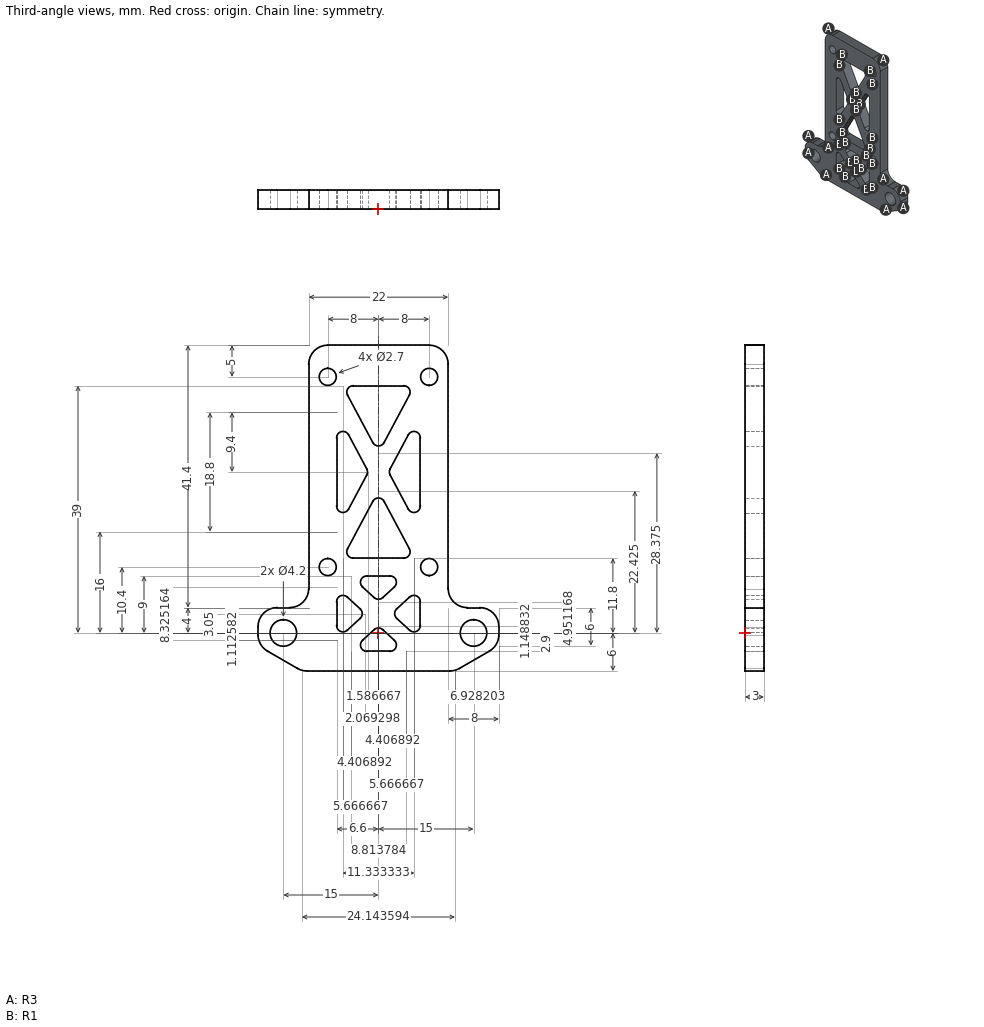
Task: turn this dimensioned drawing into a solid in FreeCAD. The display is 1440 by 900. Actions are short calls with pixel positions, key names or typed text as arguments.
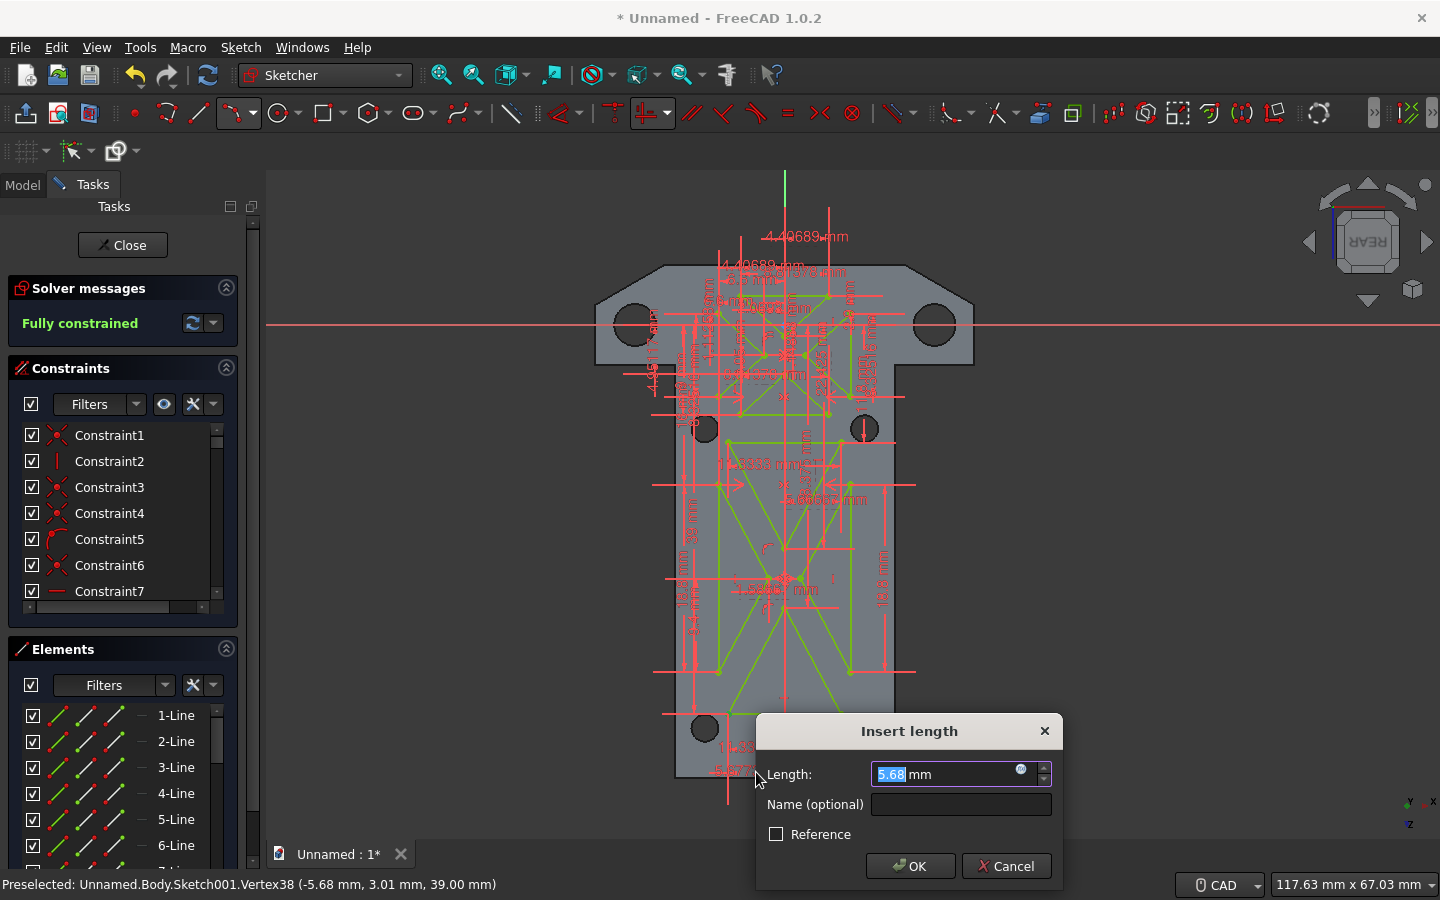
text(5.666667)
key(Return)
key(Escape)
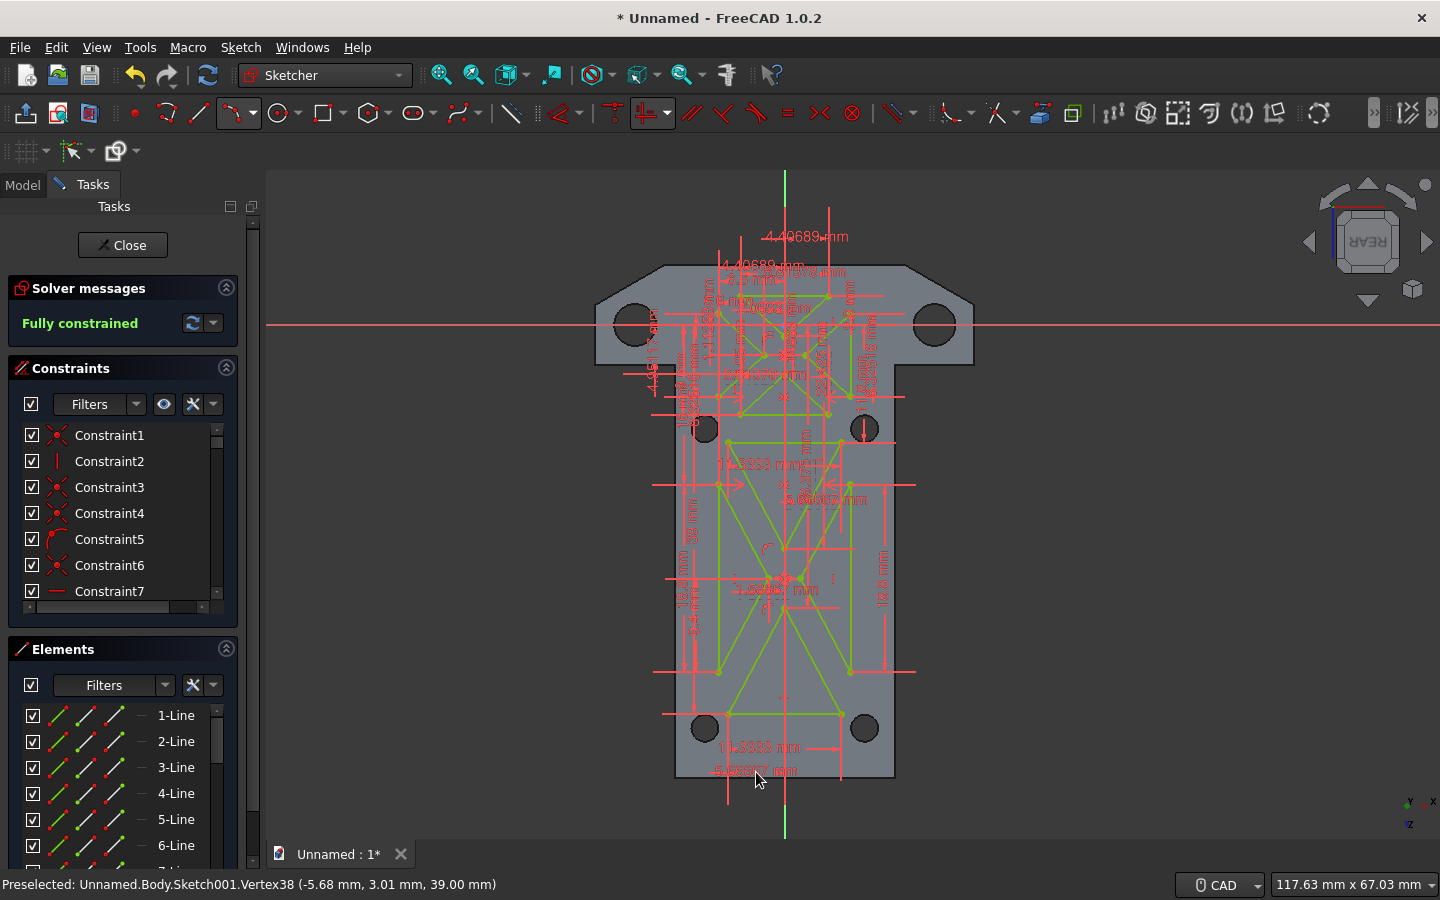
click(123, 245)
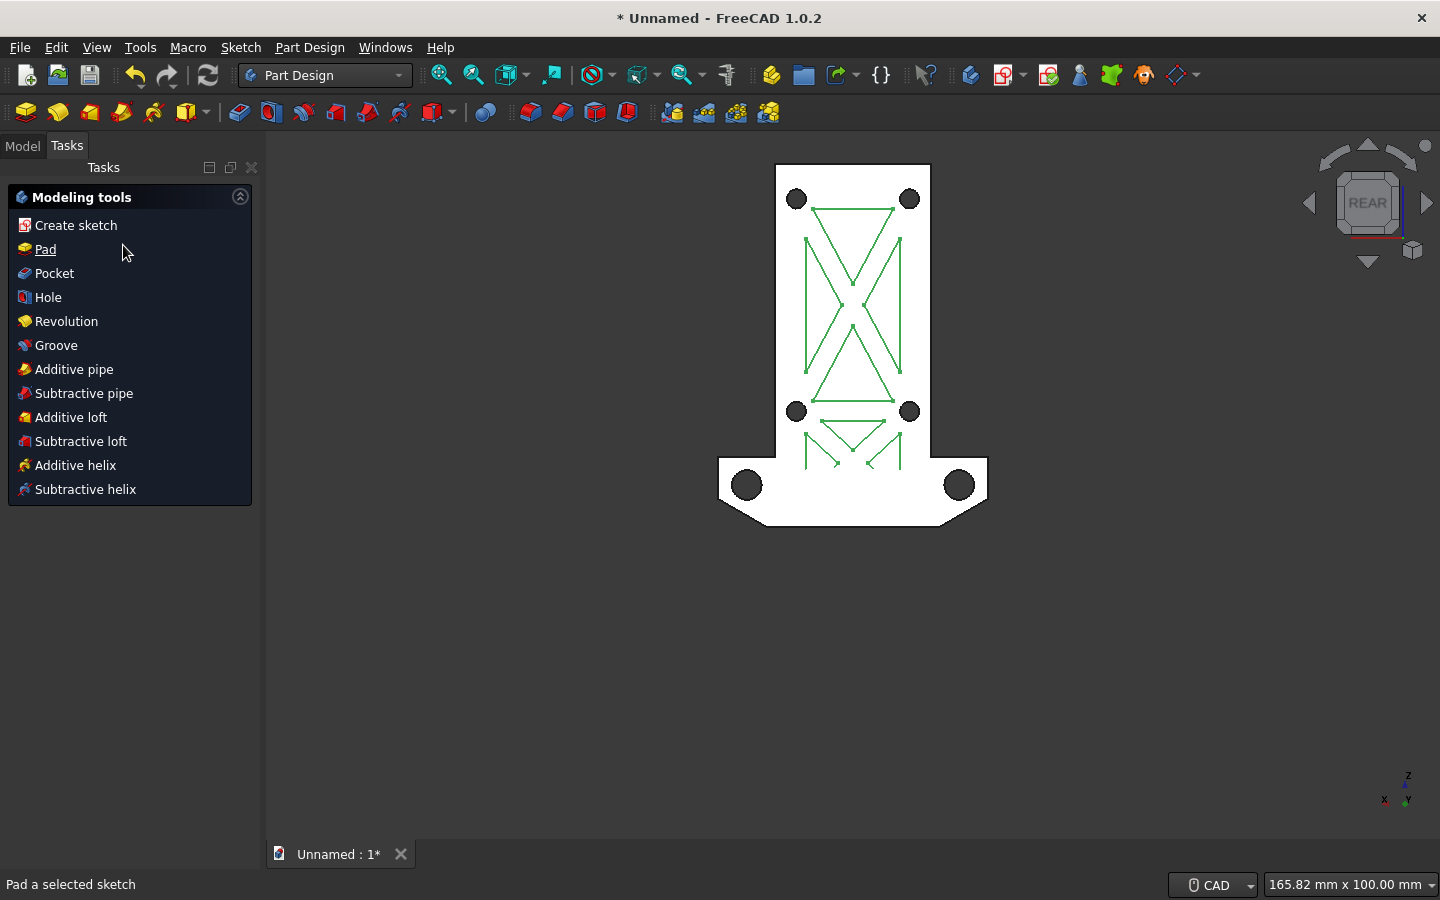
click(240, 112)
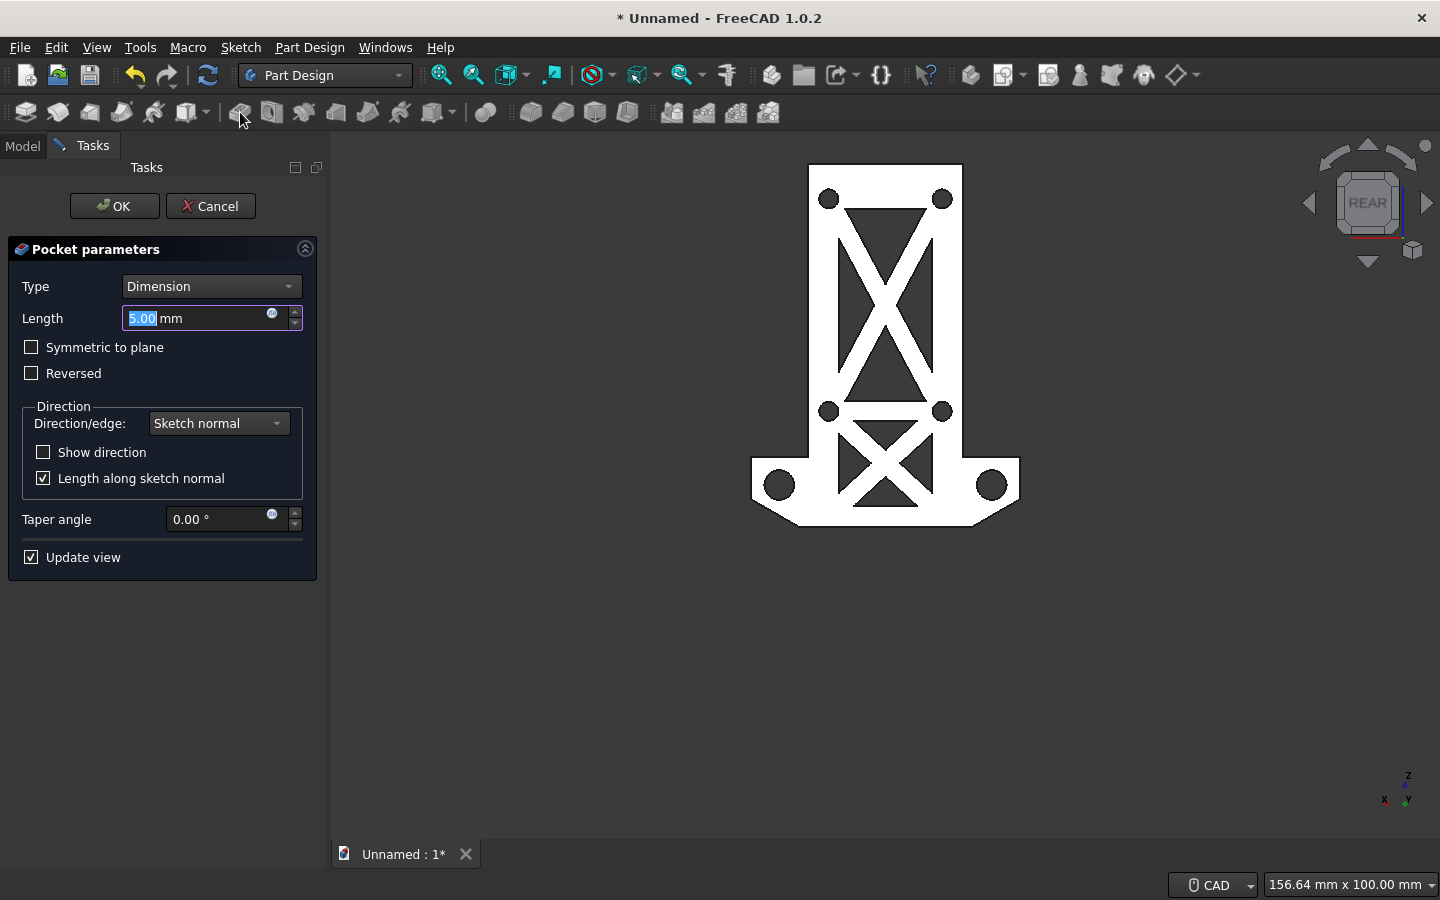
click(212, 286)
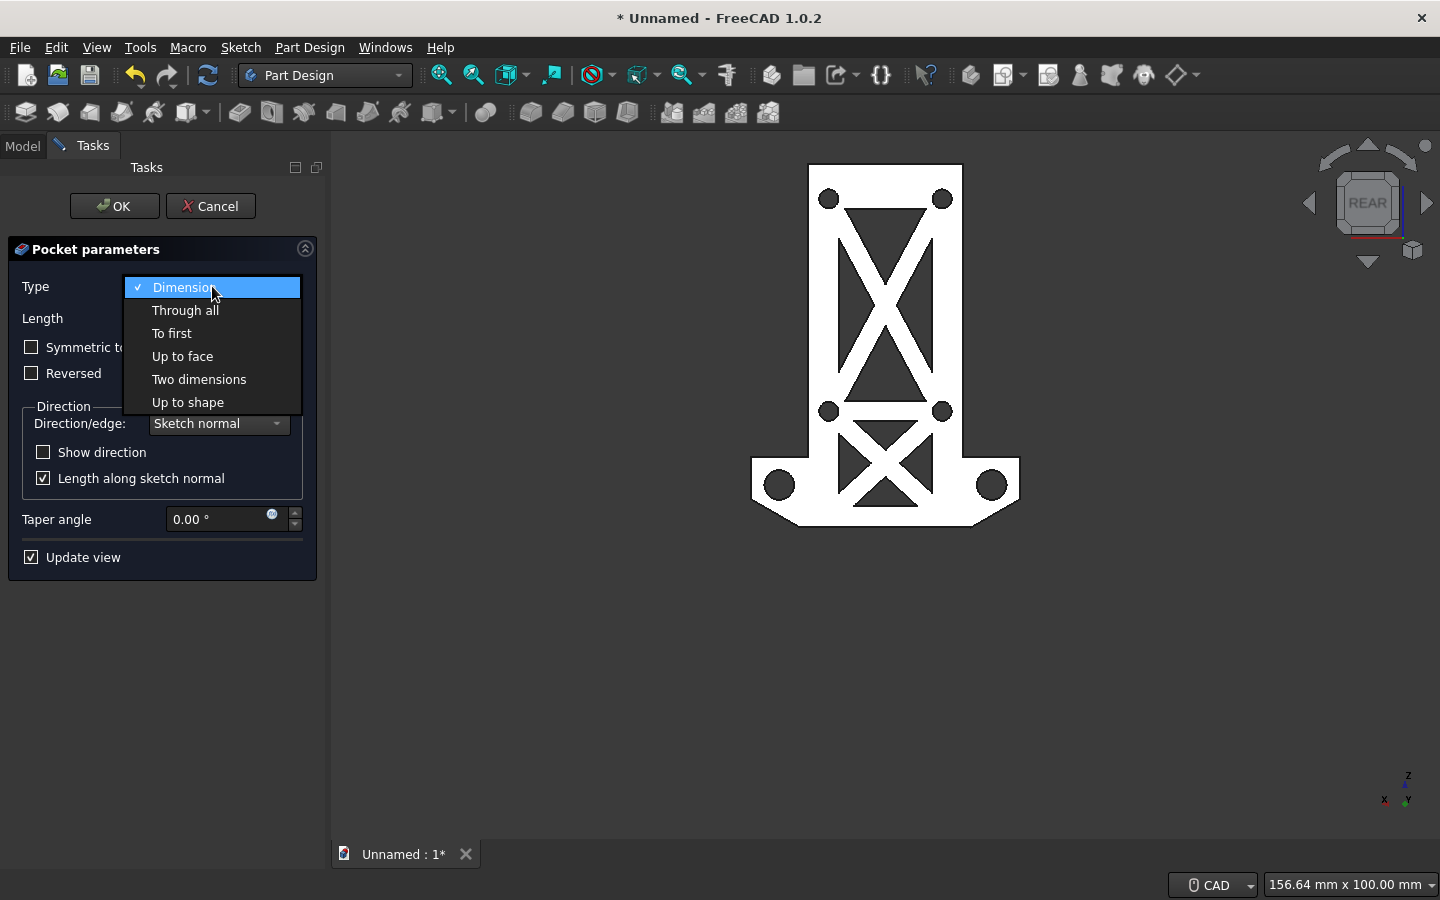
click(212, 310)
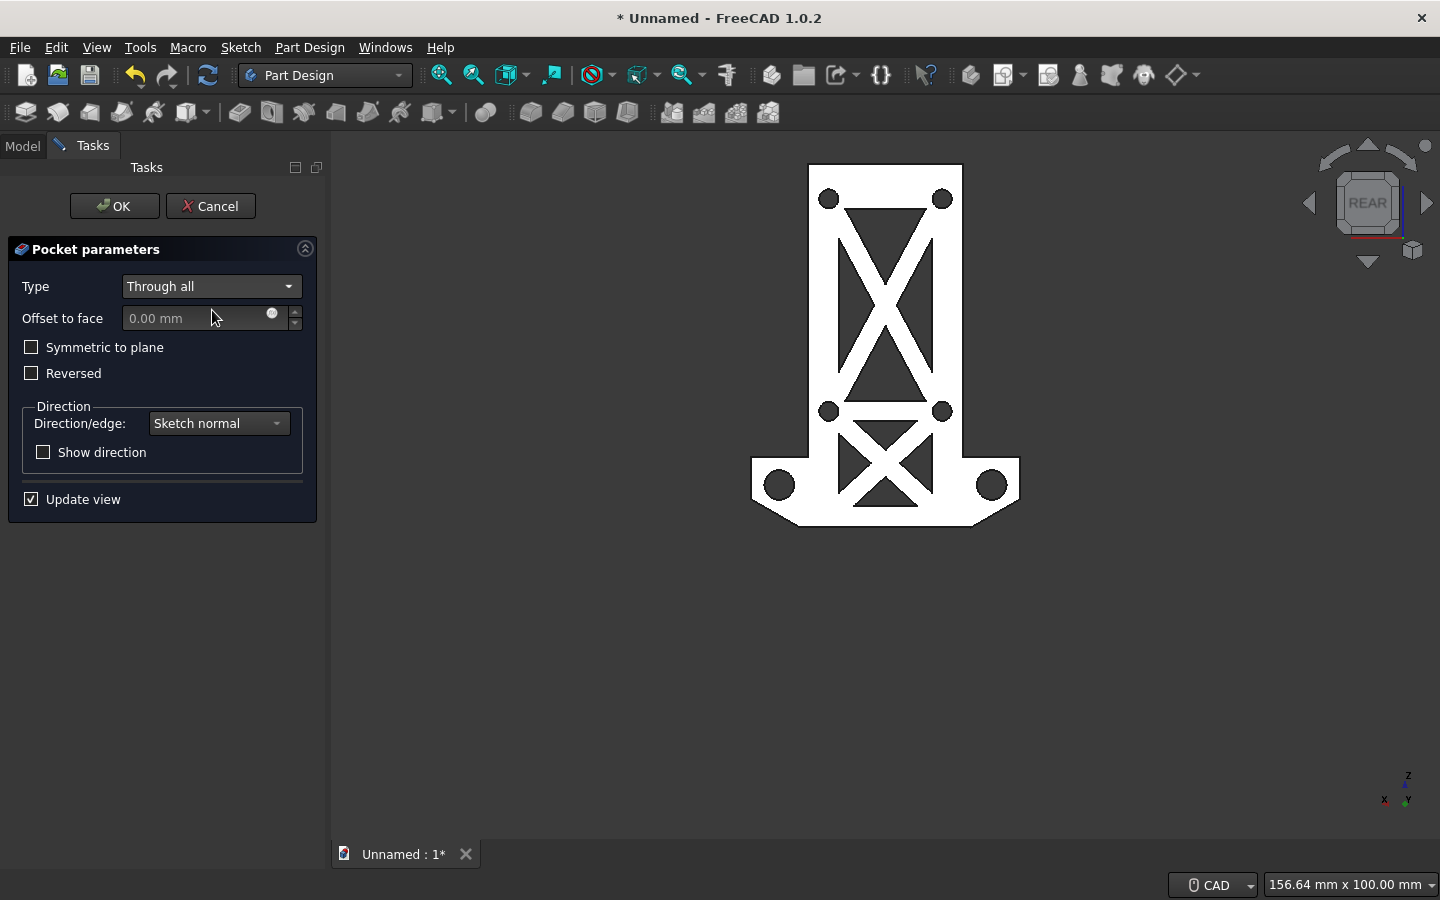
click(115, 206)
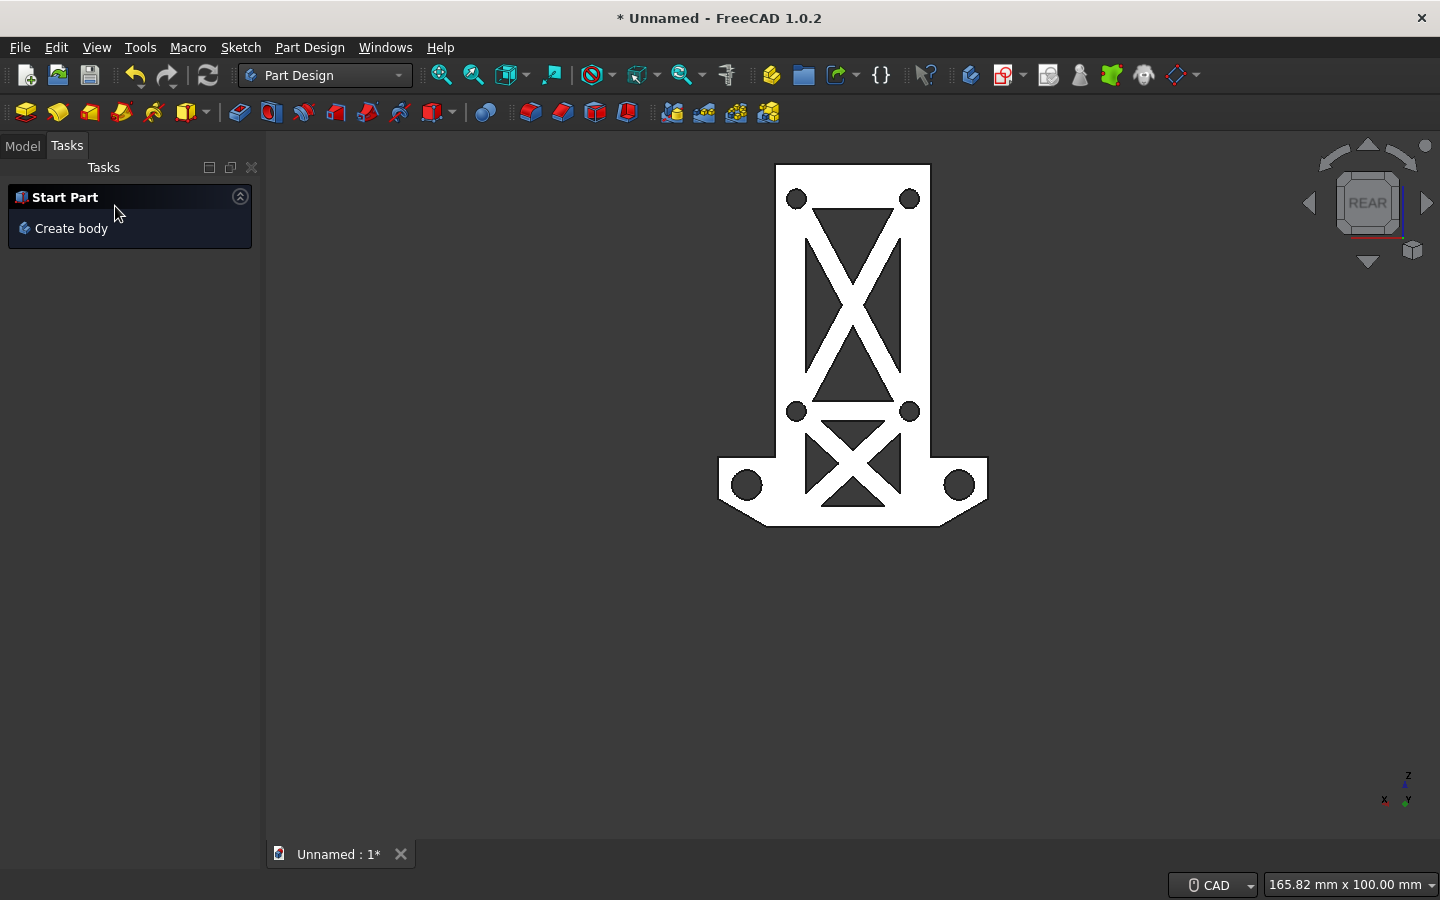
scroll(718, 456, up, 4)